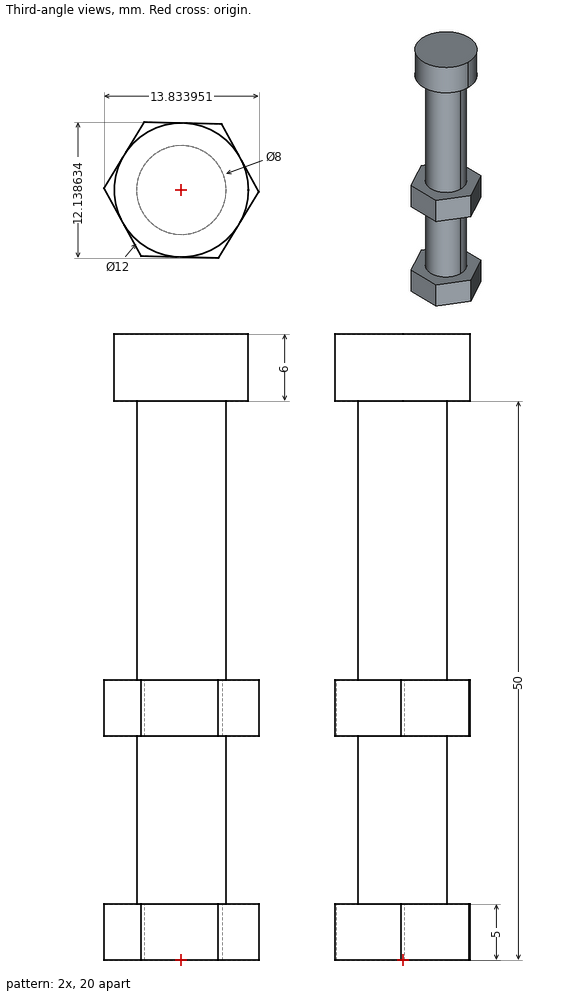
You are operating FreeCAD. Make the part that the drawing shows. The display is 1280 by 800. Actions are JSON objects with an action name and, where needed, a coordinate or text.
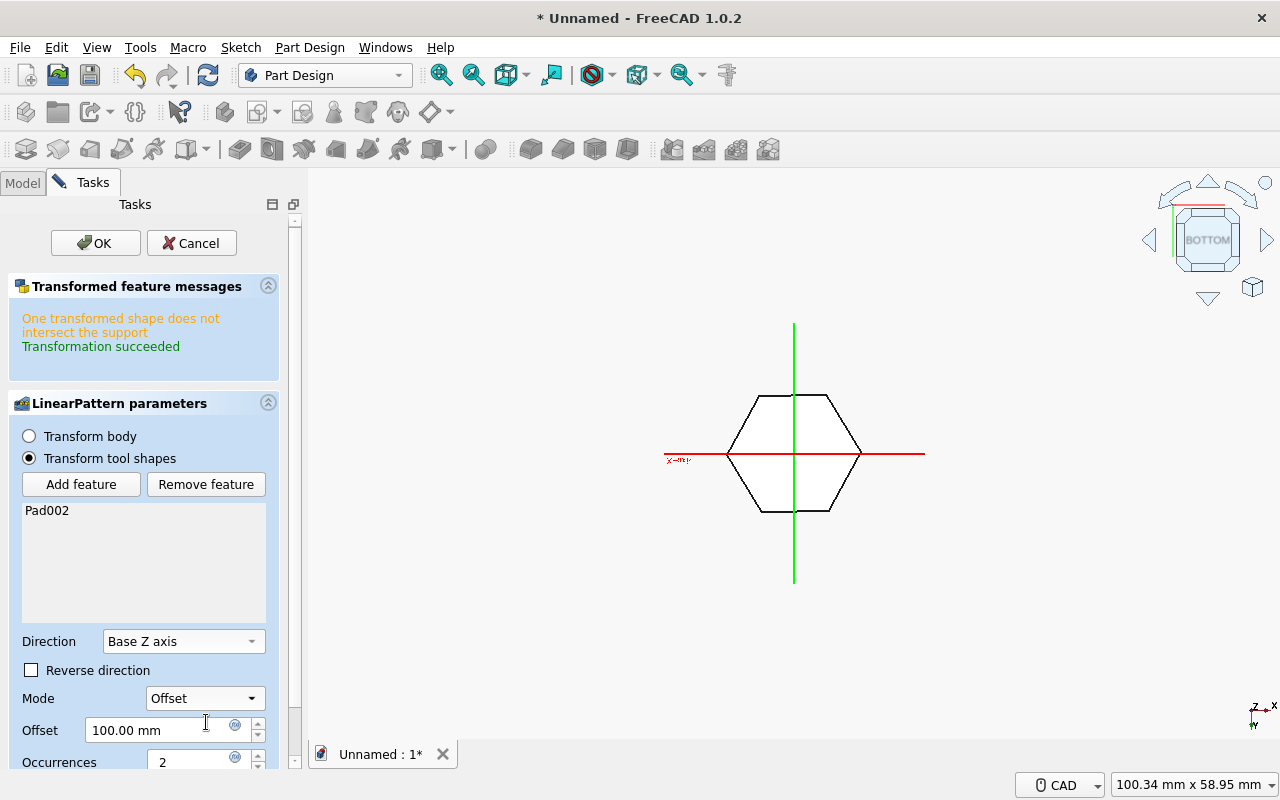
{"action": "triple_click", "coordinate": [168, 730]}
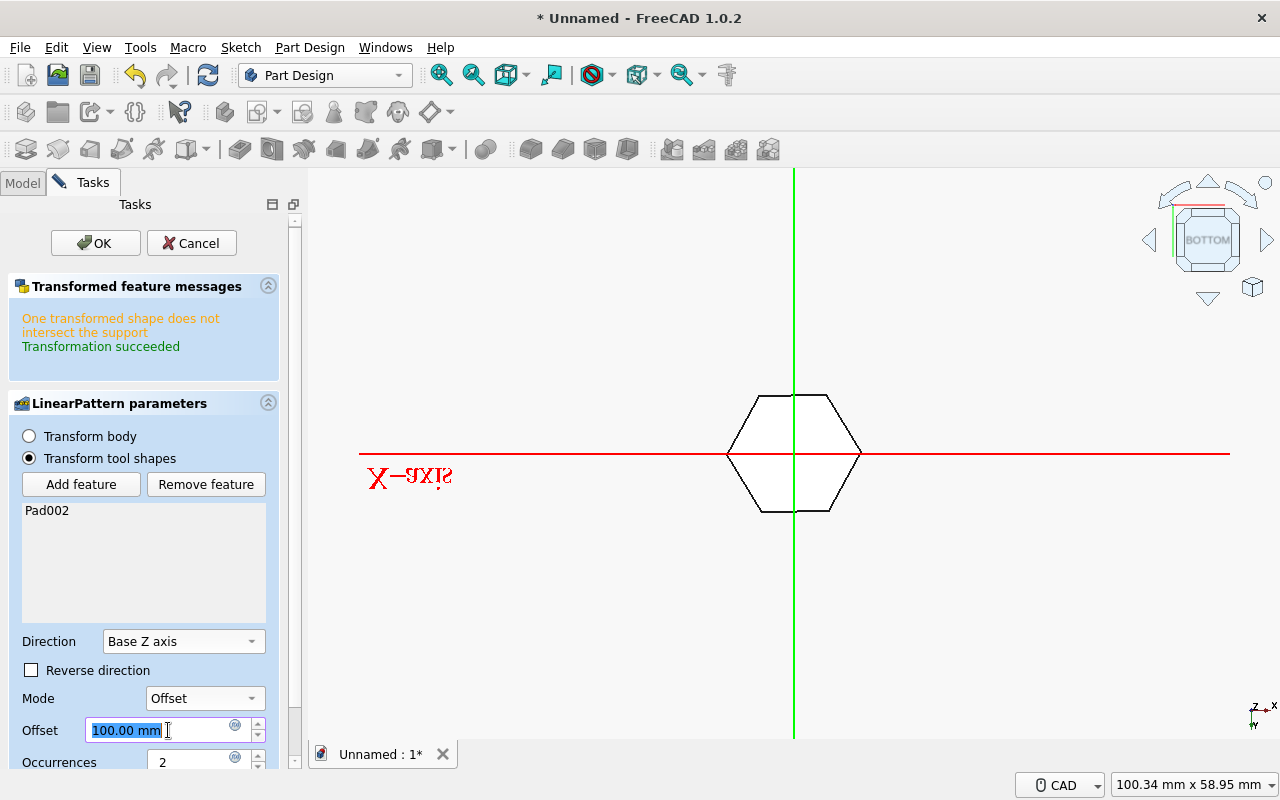
{"action": "type", "text": "20"}
{"action": "key", "text": "Tab"}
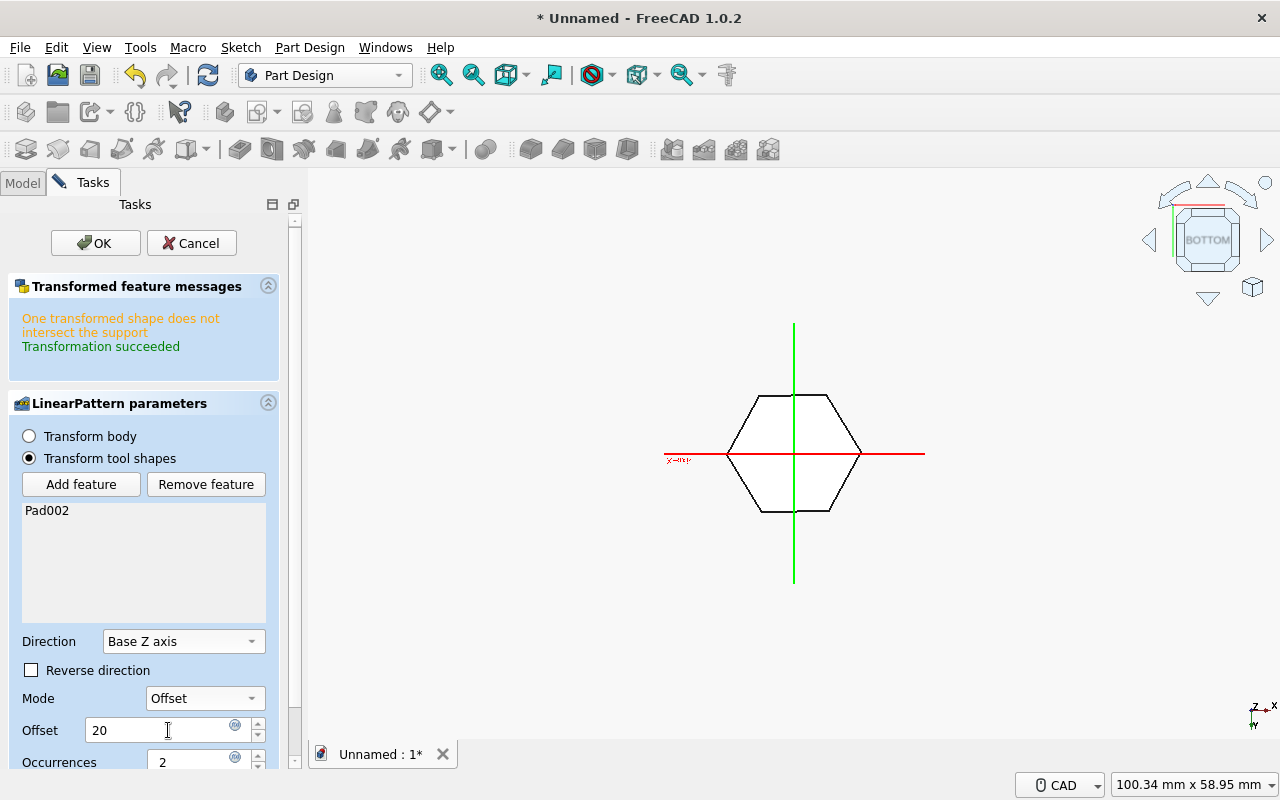
{"action": "scroll", "coordinate": [295, 491], "scroll_direction": "down", "scroll_amount": 2}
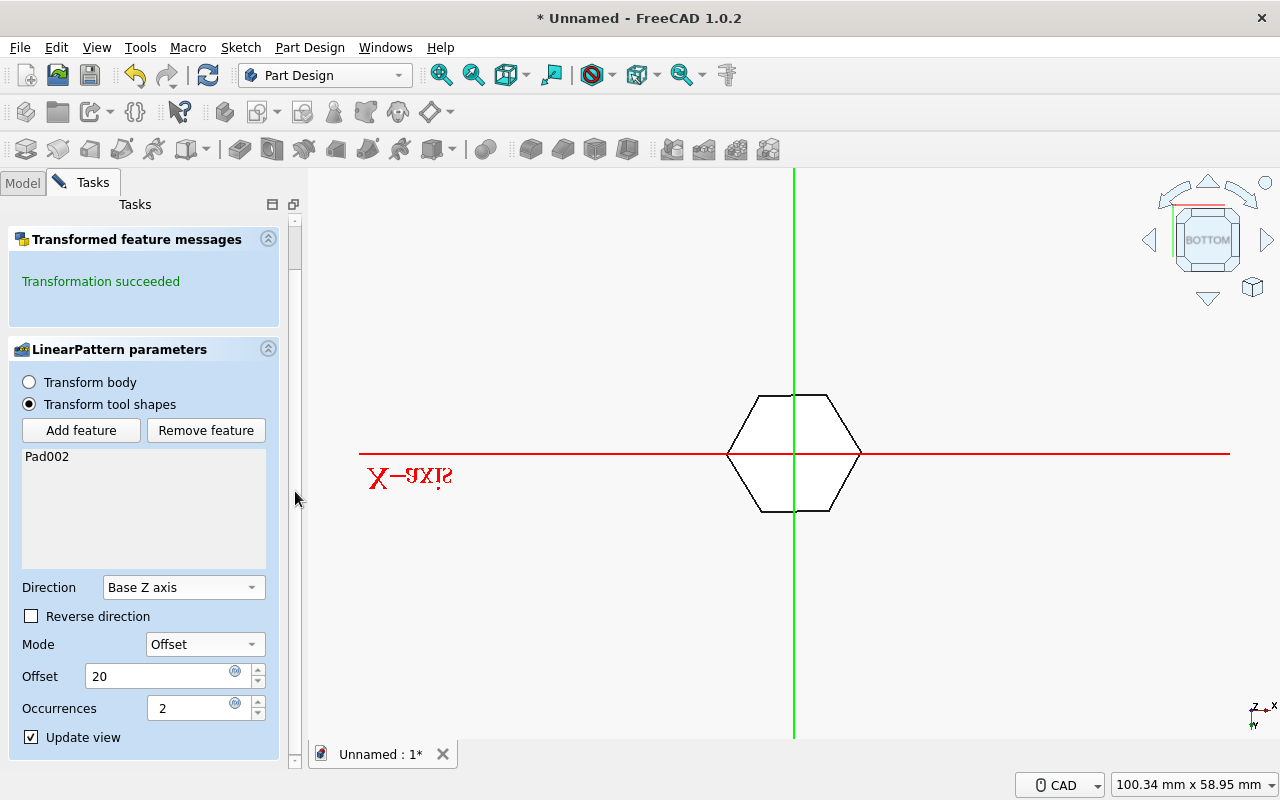
{"action": "triple_click", "coordinate": [198, 708]}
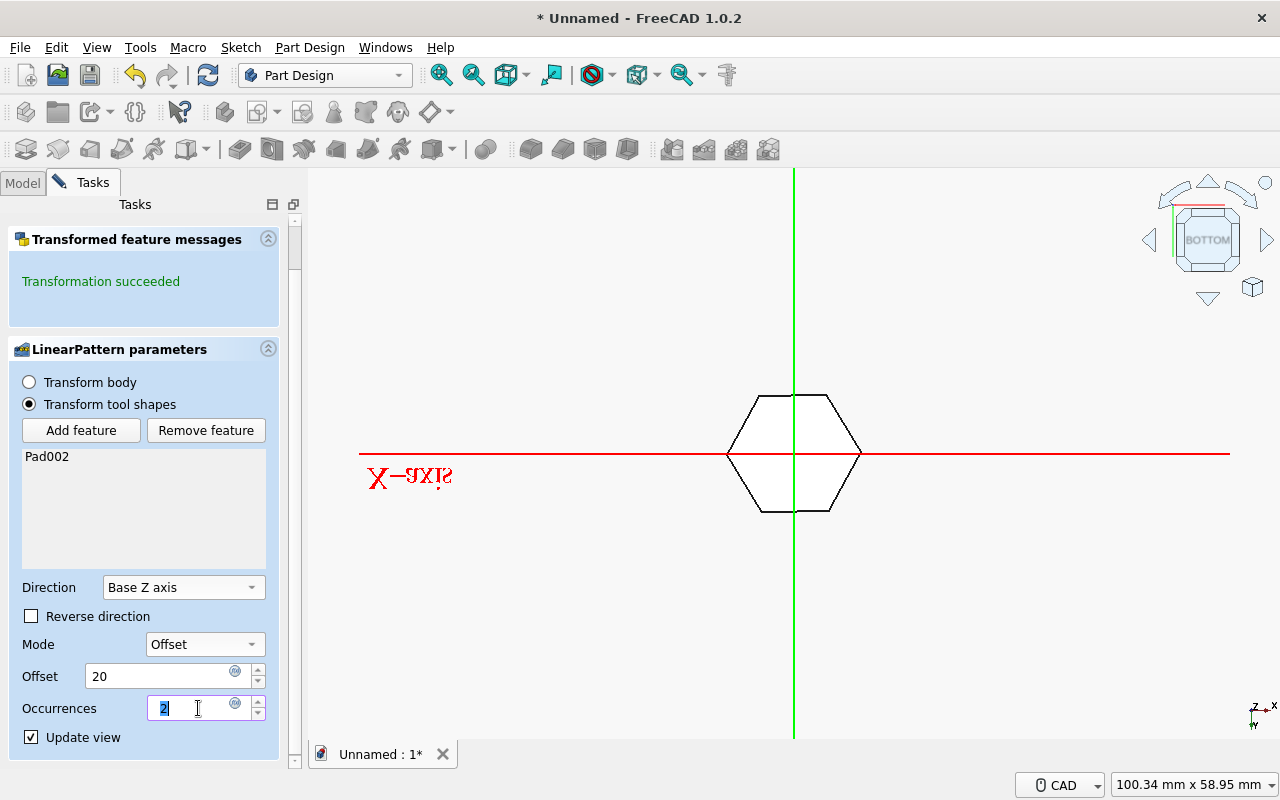
{"action": "type", "text": "2"}
{"action": "key", "text": "Tab"}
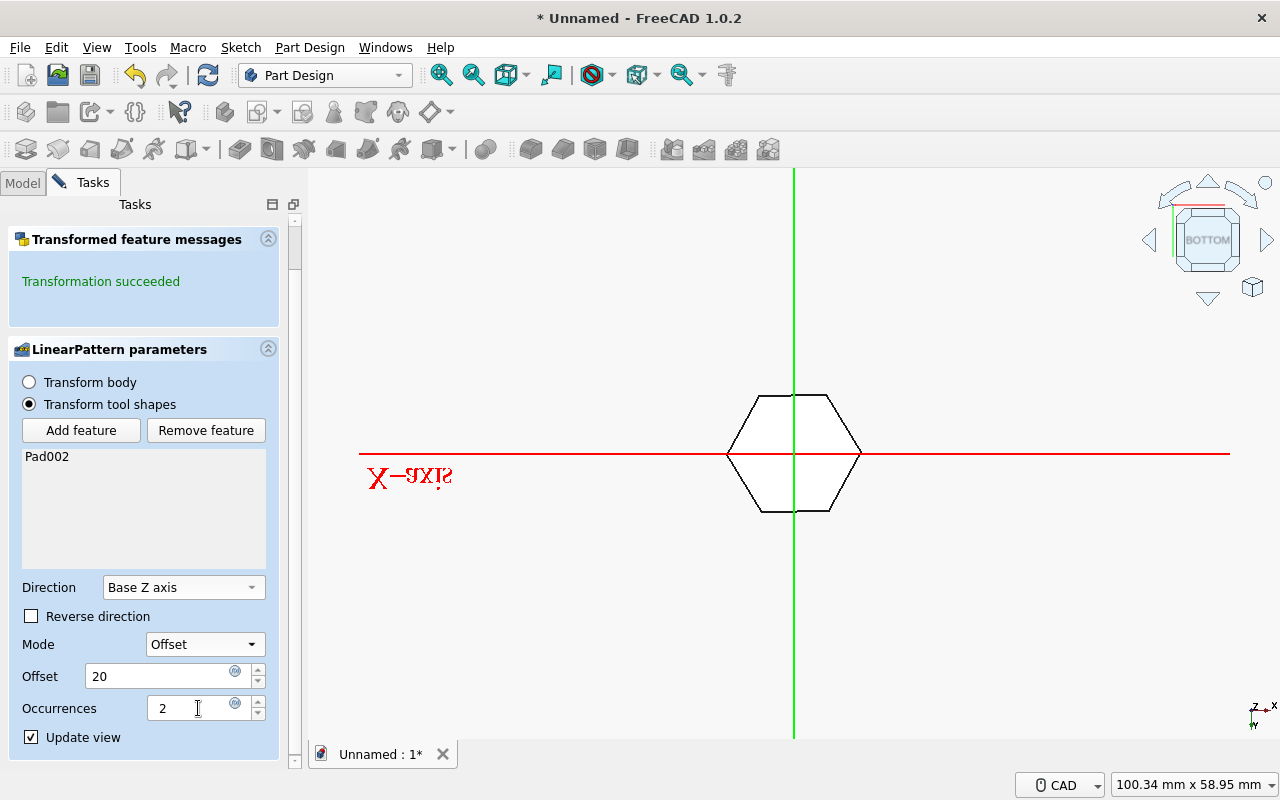
{"action": "scroll", "coordinate": [295, 491], "scroll_direction": "up", "scroll_amount": 2}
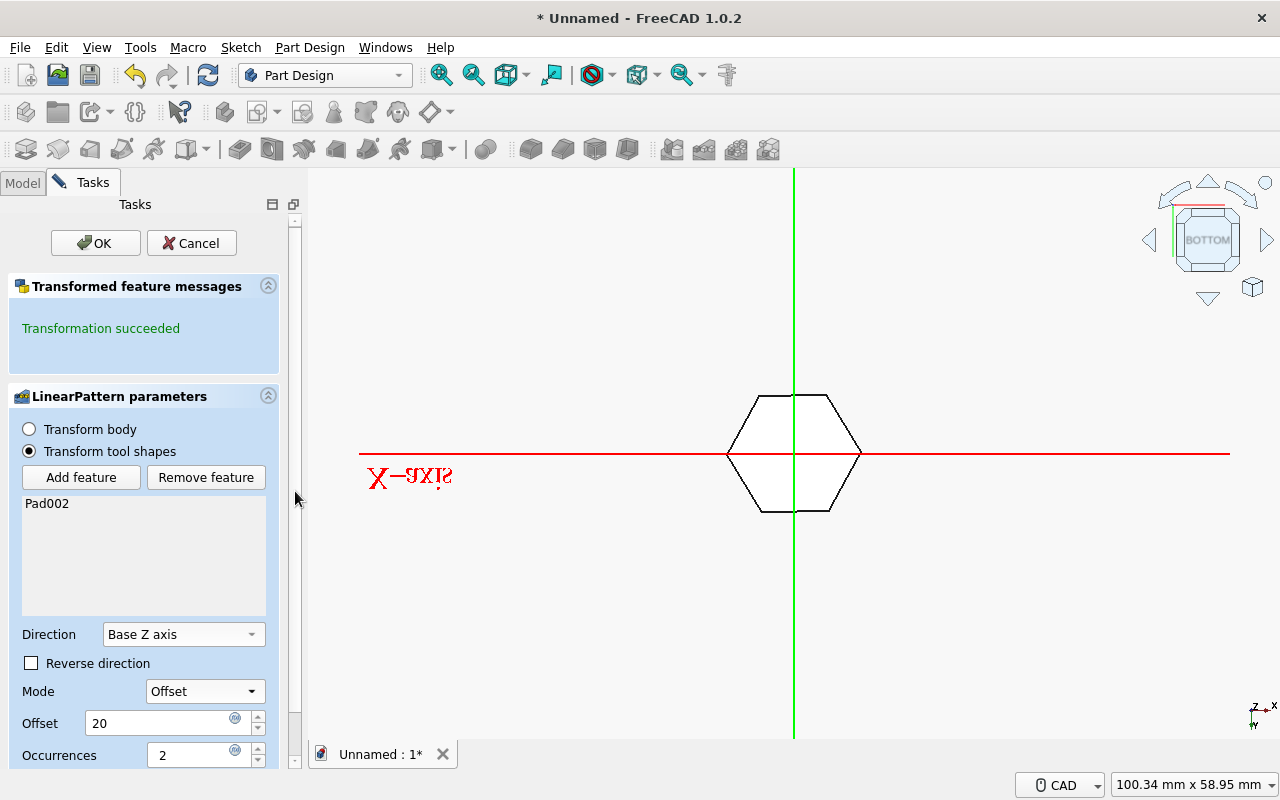
{"action": "left_click", "coordinate": [96, 243]}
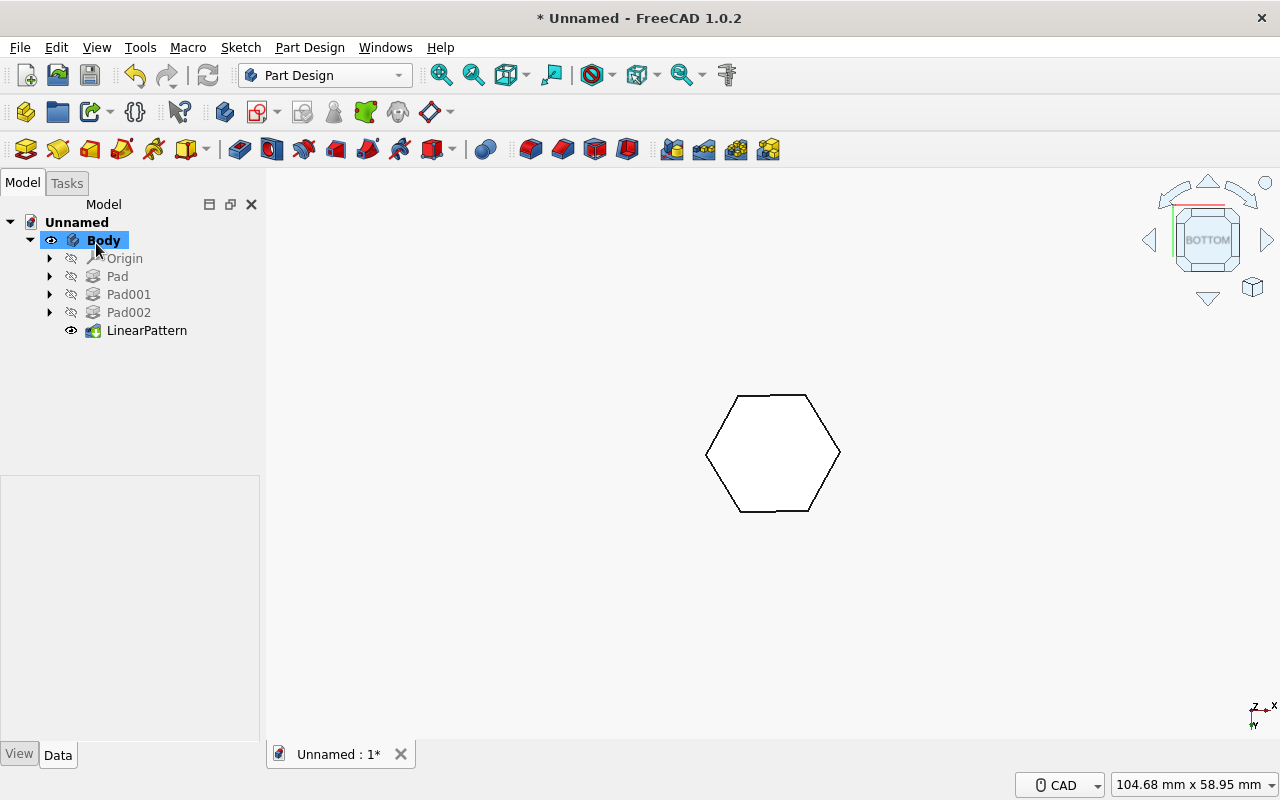
{"action": "key", "text": "0"}